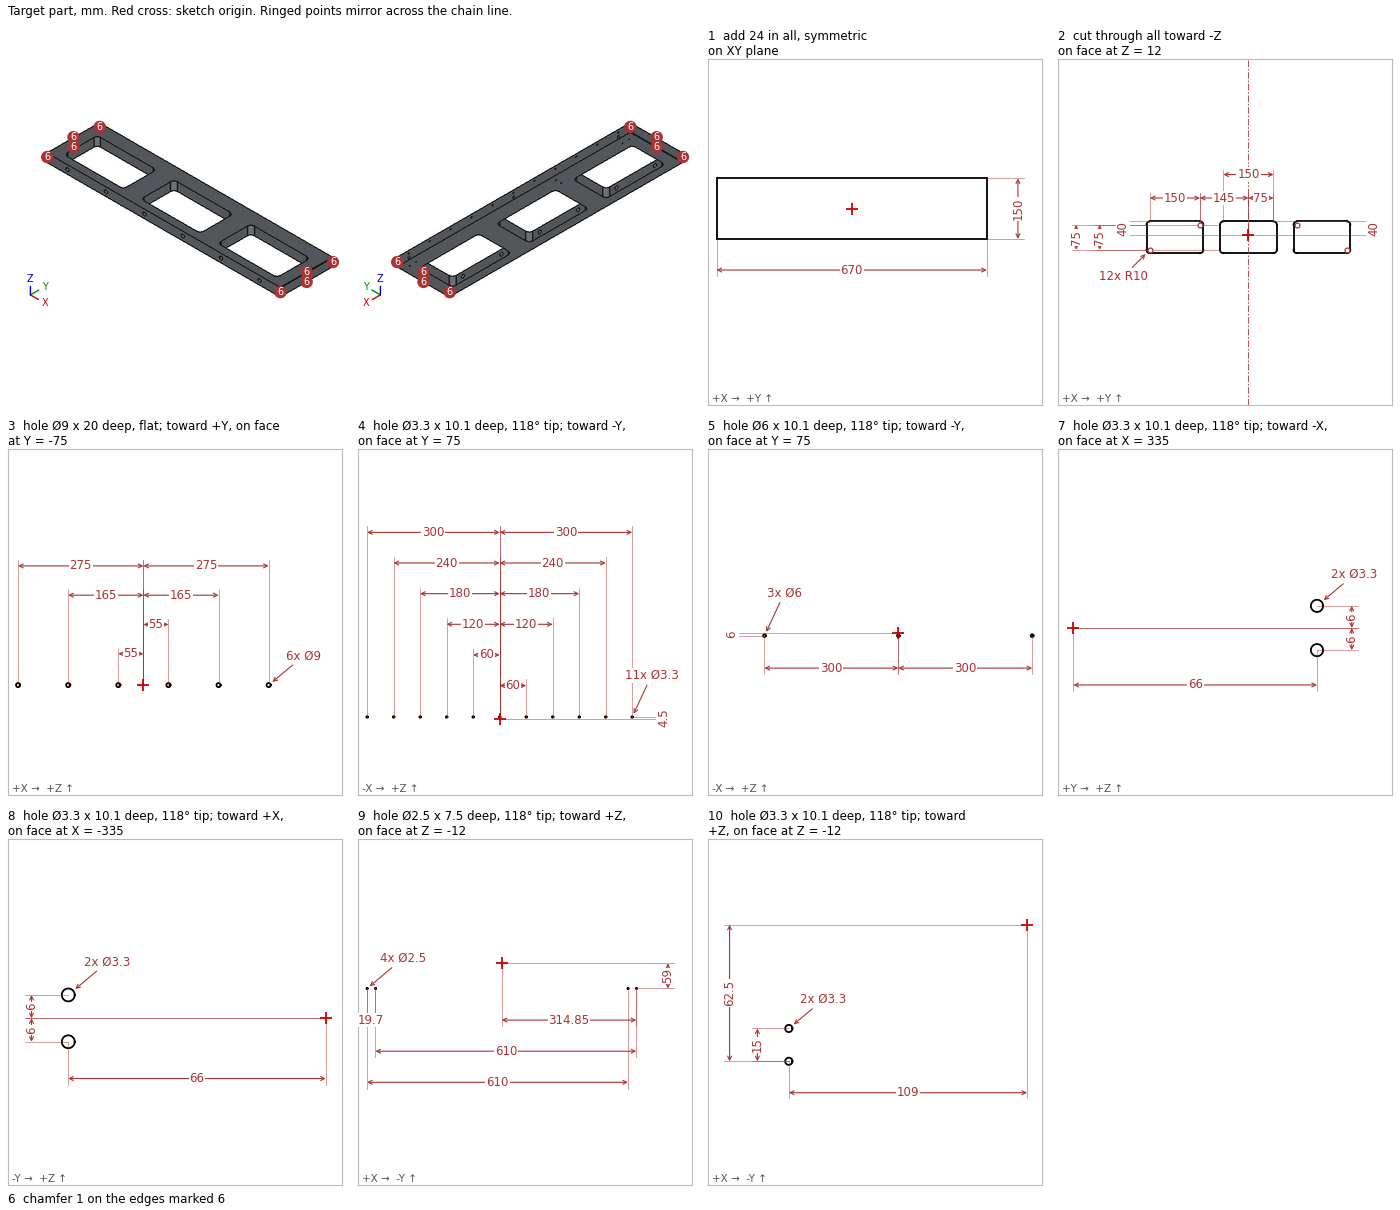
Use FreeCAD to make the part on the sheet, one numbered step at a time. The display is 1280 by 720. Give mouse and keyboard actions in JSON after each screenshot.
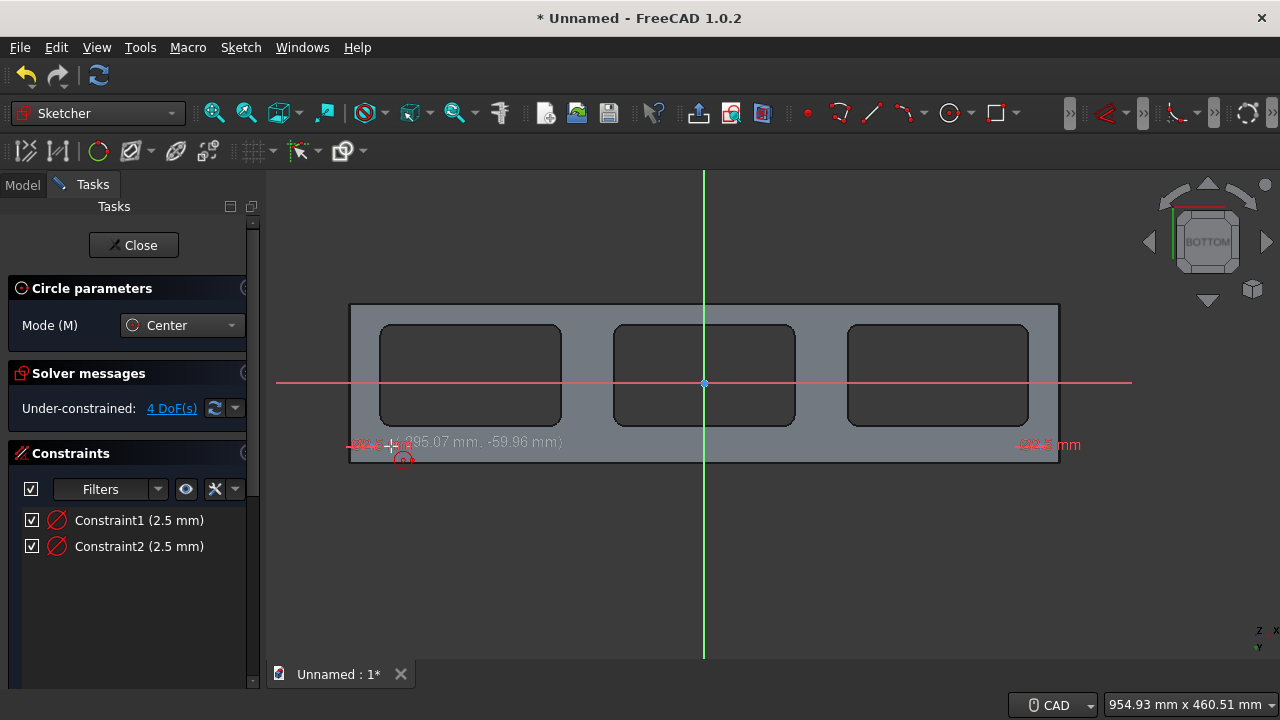
{"action": "left_click", "coordinate": [391, 446]}
{"action": "mouse_move", "coordinate": [392, 445]}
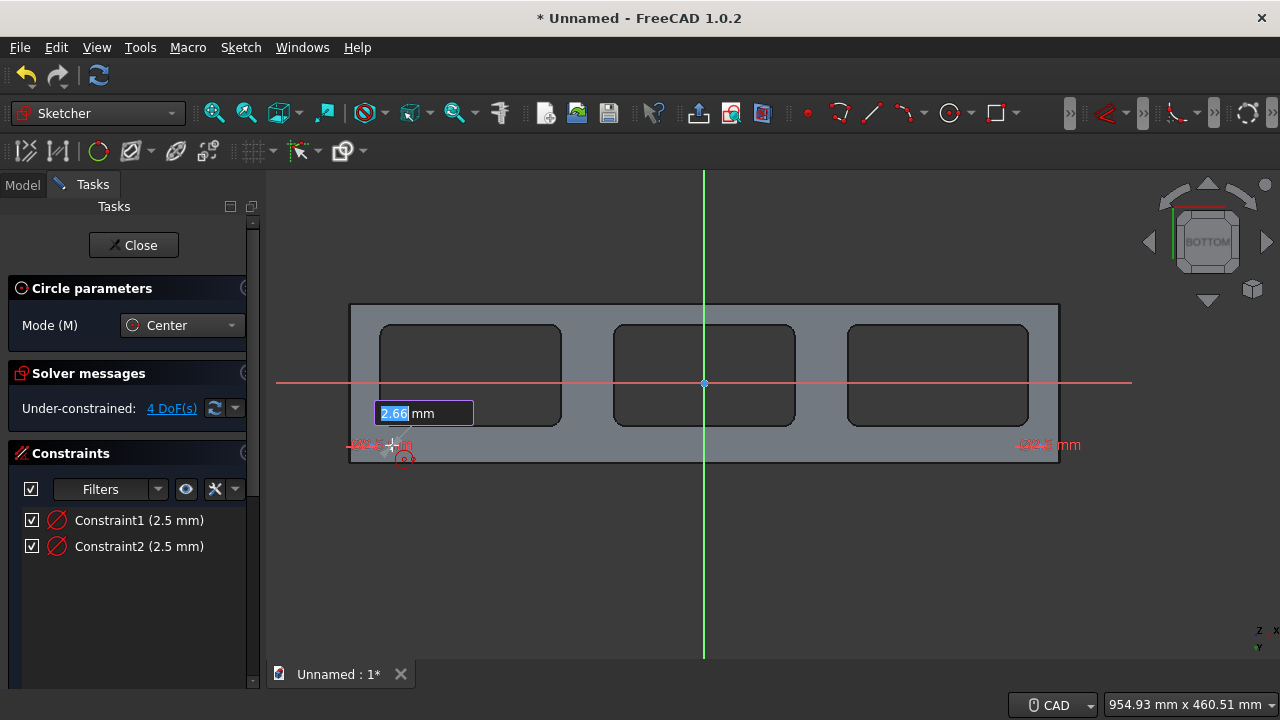
{"action": "type", "text": "2.5"}
{"action": "key", "text": "Return"}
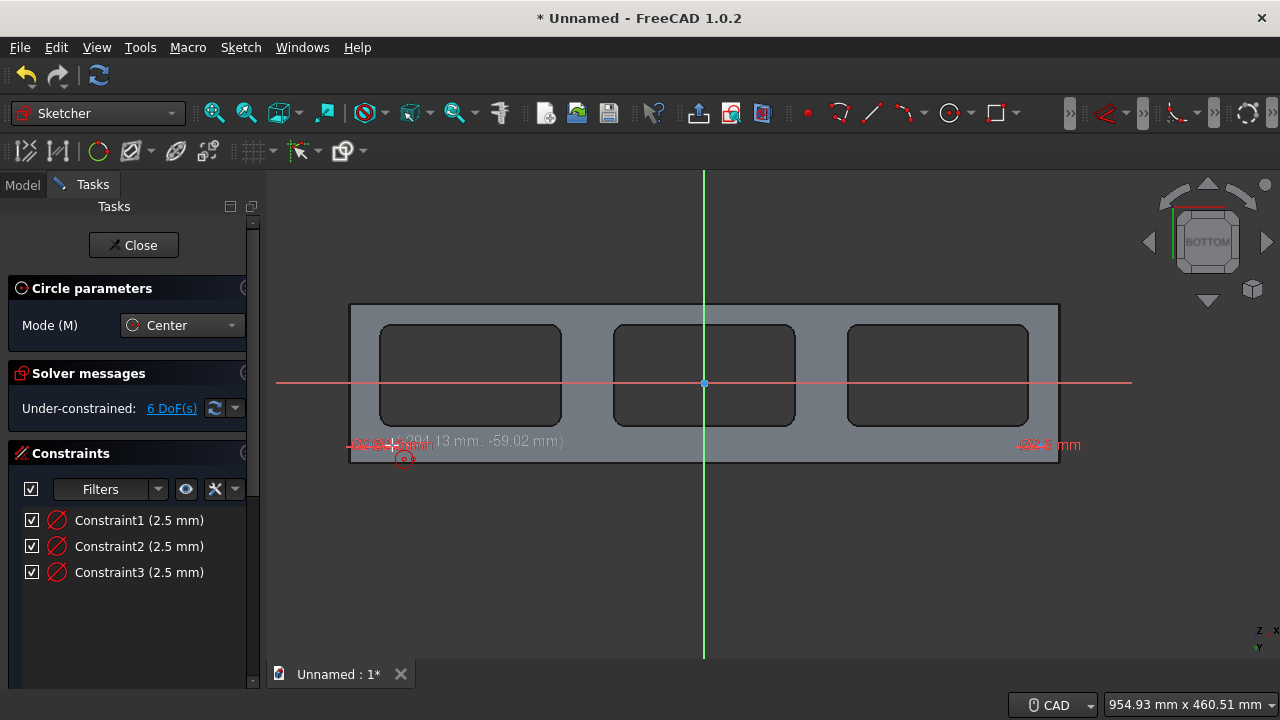
{"action": "scroll", "coordinate": [1018, 446], "scroll_direction": "up", "scroll_amount": 15}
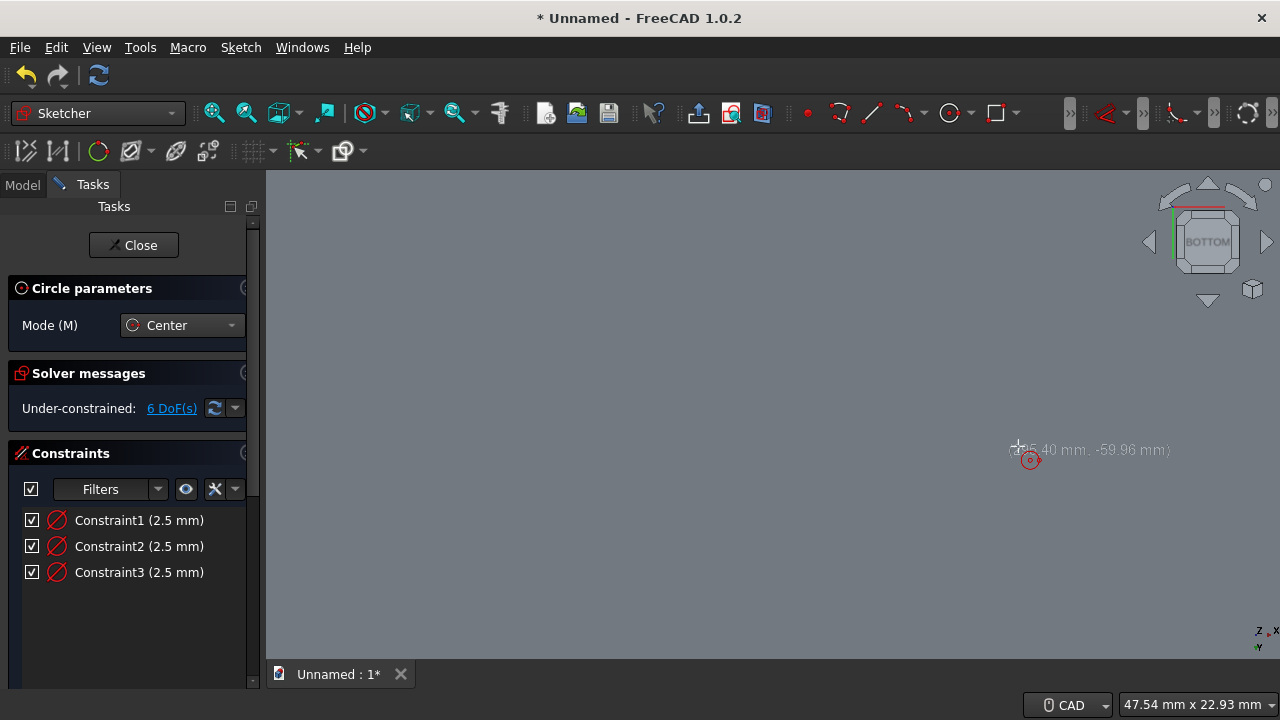
{"action": "scroll", "coordinate": [1019, 446], "scroll_direction": "down", "scroll_amount": 15}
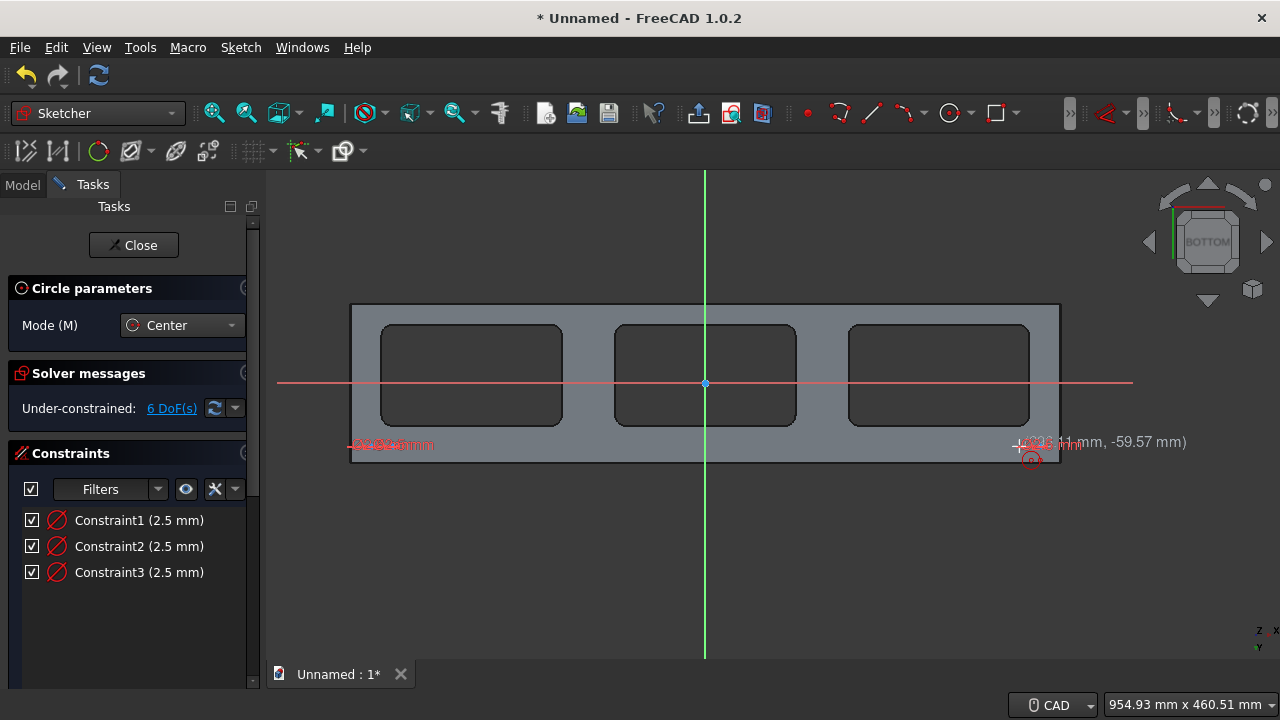
{"action": "left_click", "coordinate": [1019, 446]}
{"action": "mouse_move", "coordinate": [1020, 445]}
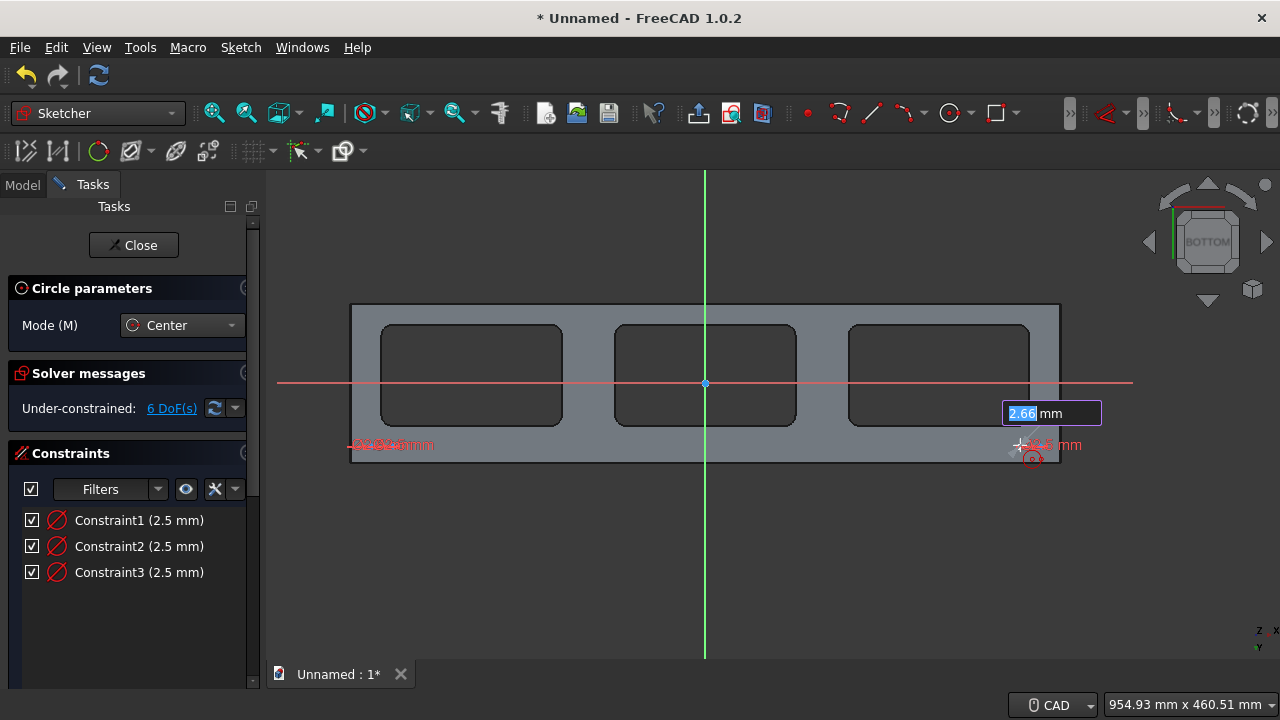
{"action": "type", "text": "2.5"}
{"action": "key", "text": "Return"}
{"action": "key", "text": "Escape"}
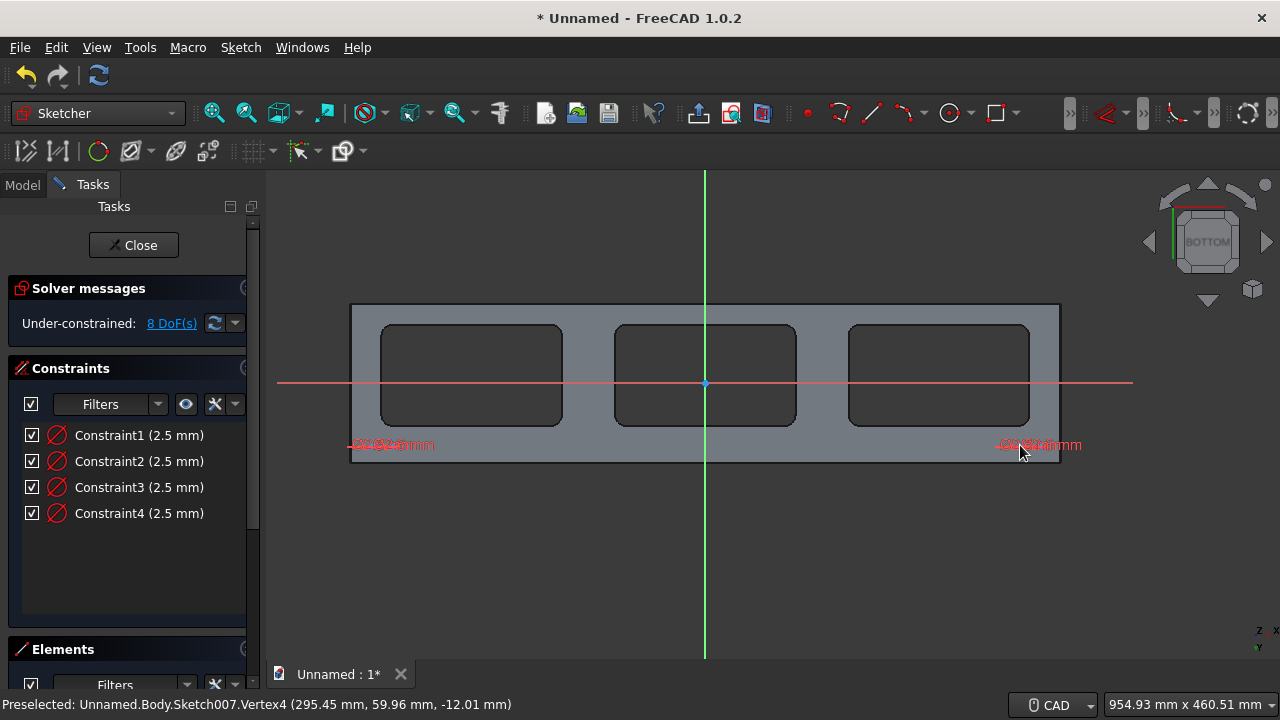
{"action": "left_click", "coordinate": [1040, 447]}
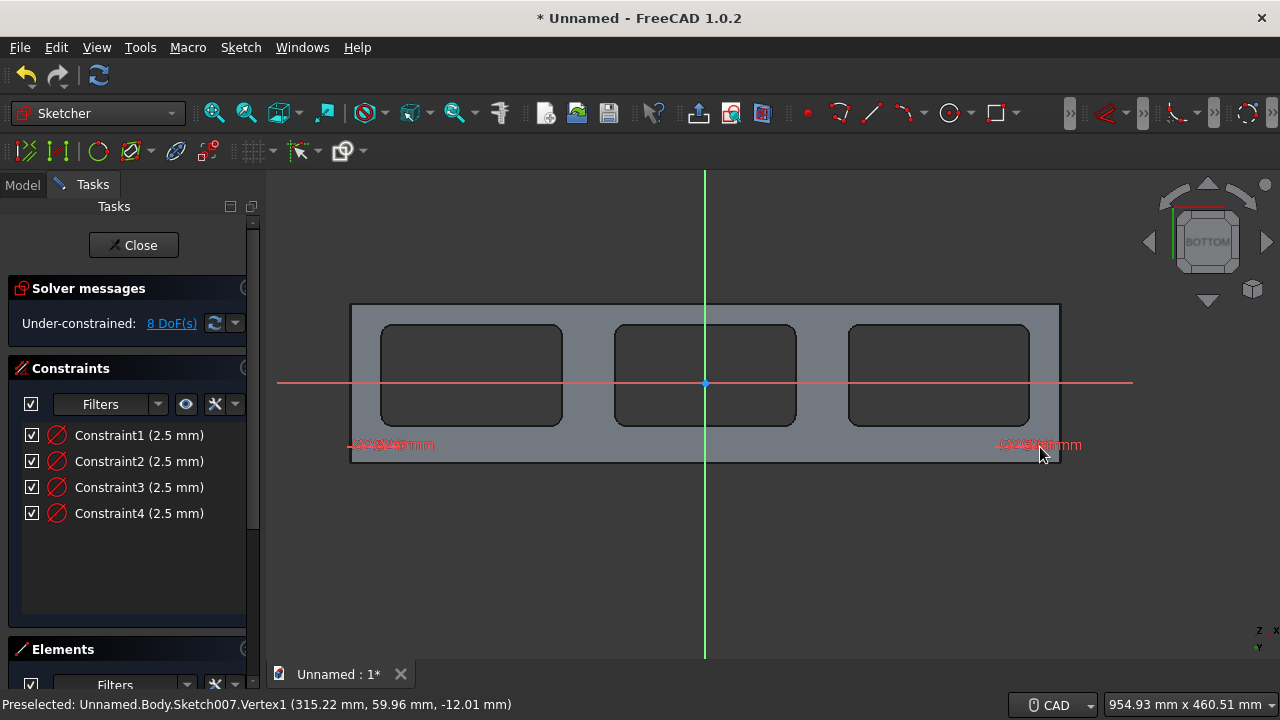
{"action": "left_click", "coordinate": [371, 447]}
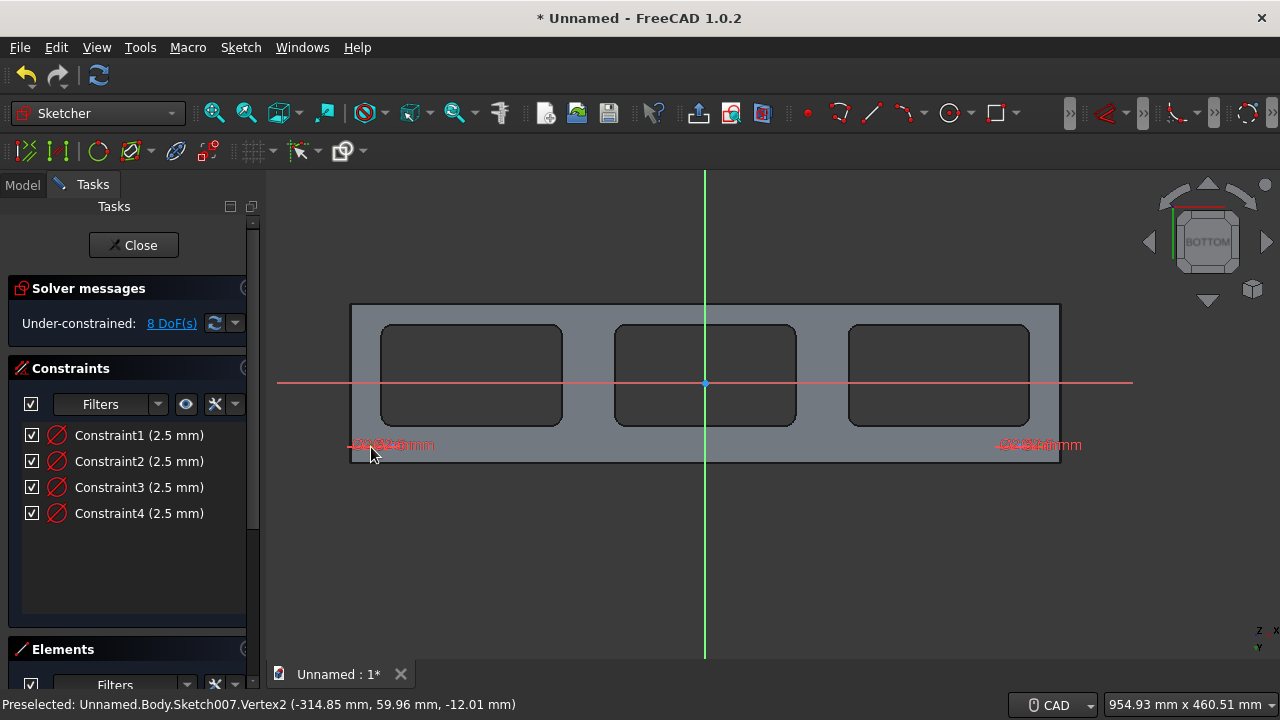
{"action": "key", "text": "h"}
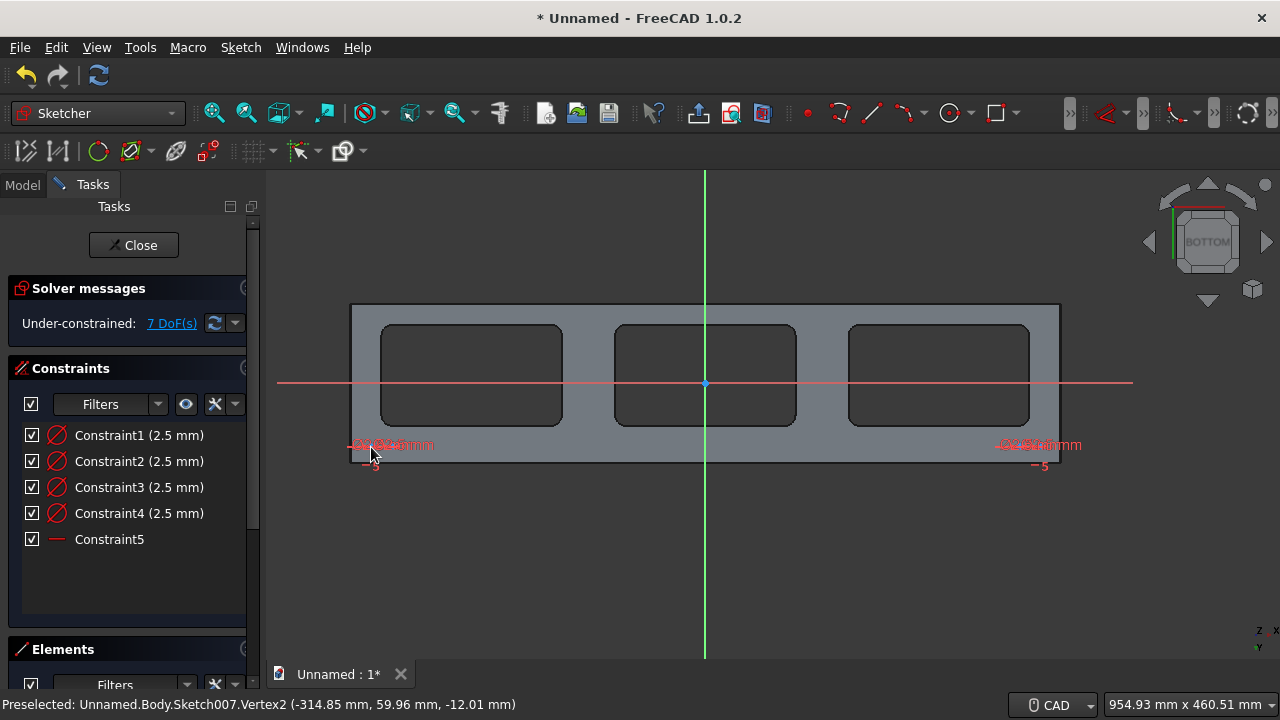
{"action": "left_click", "coordinate": [371, 447]}